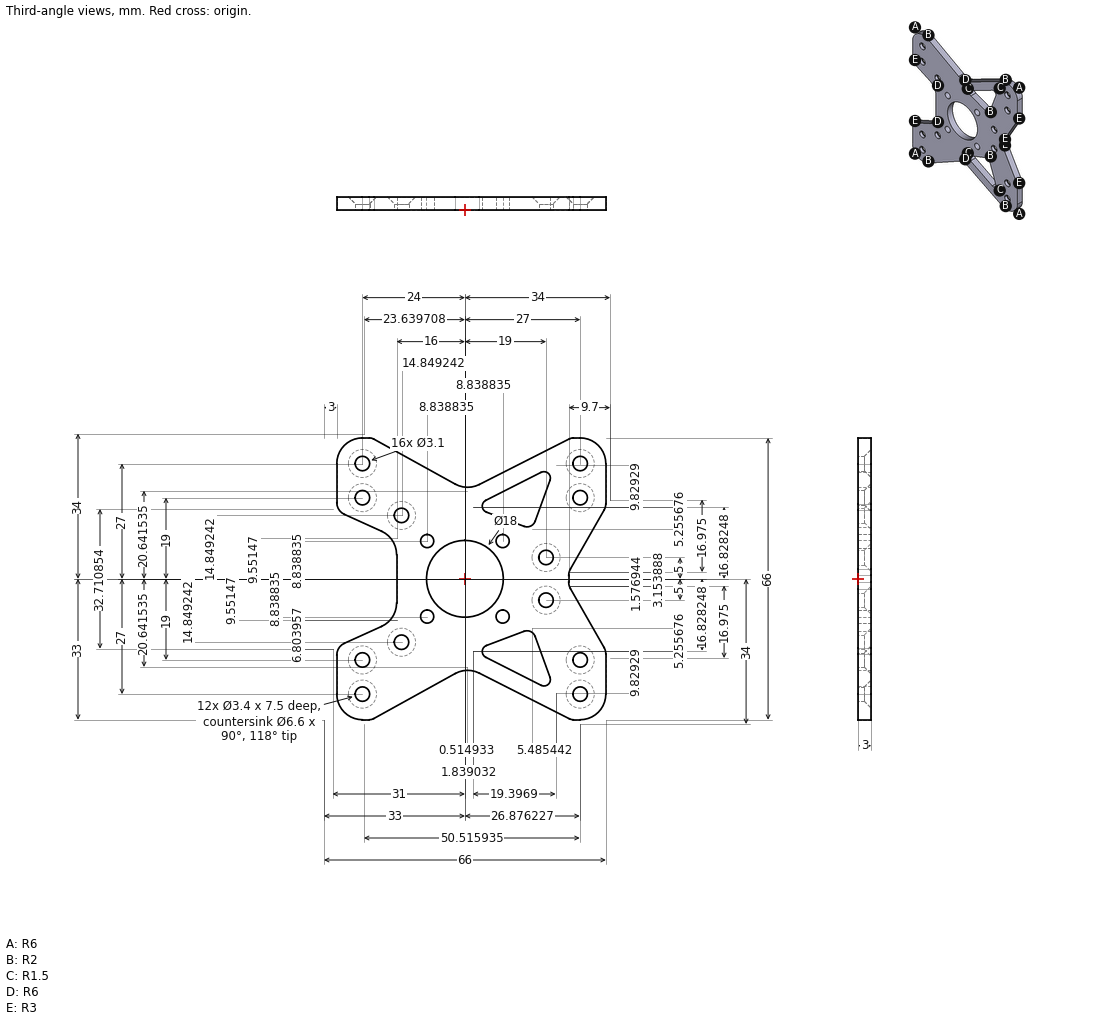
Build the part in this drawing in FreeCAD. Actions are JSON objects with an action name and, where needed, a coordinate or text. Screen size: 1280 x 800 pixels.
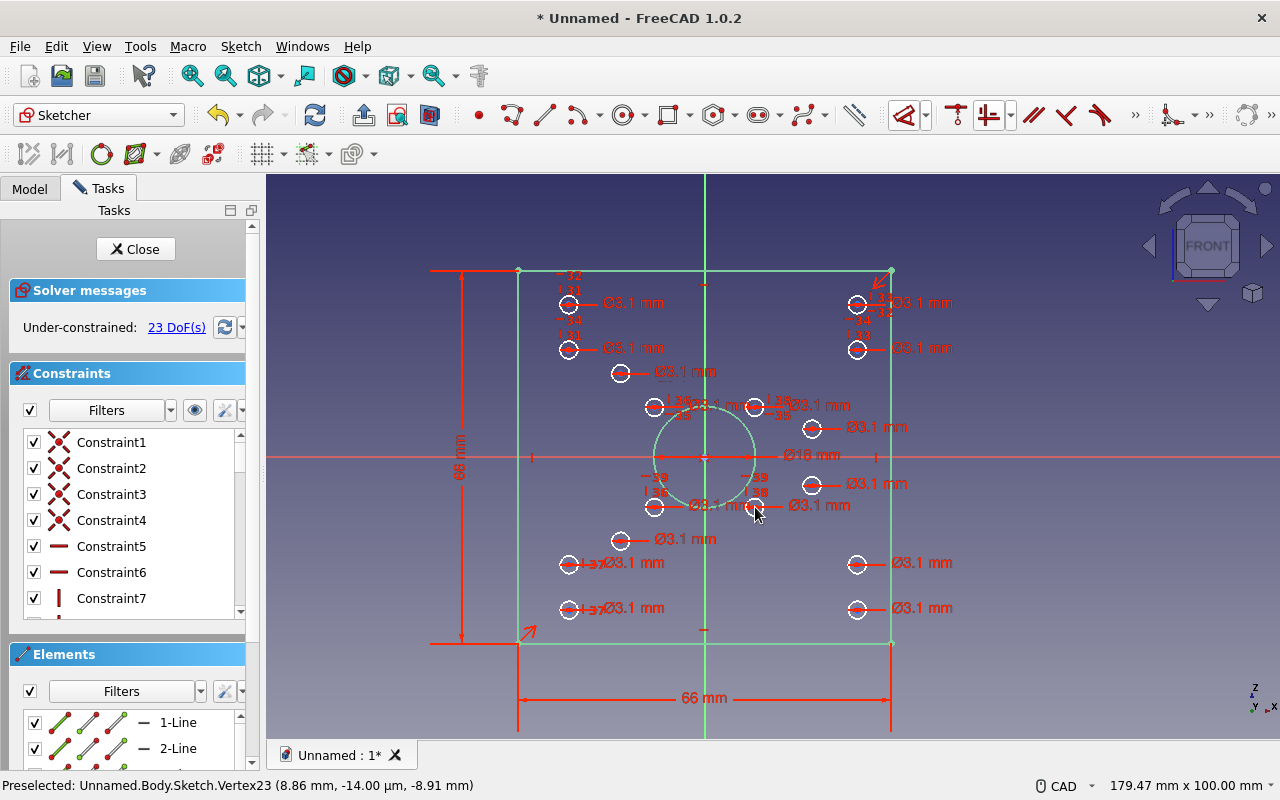
{"action": "left_click", "coordinate": [812, 429]}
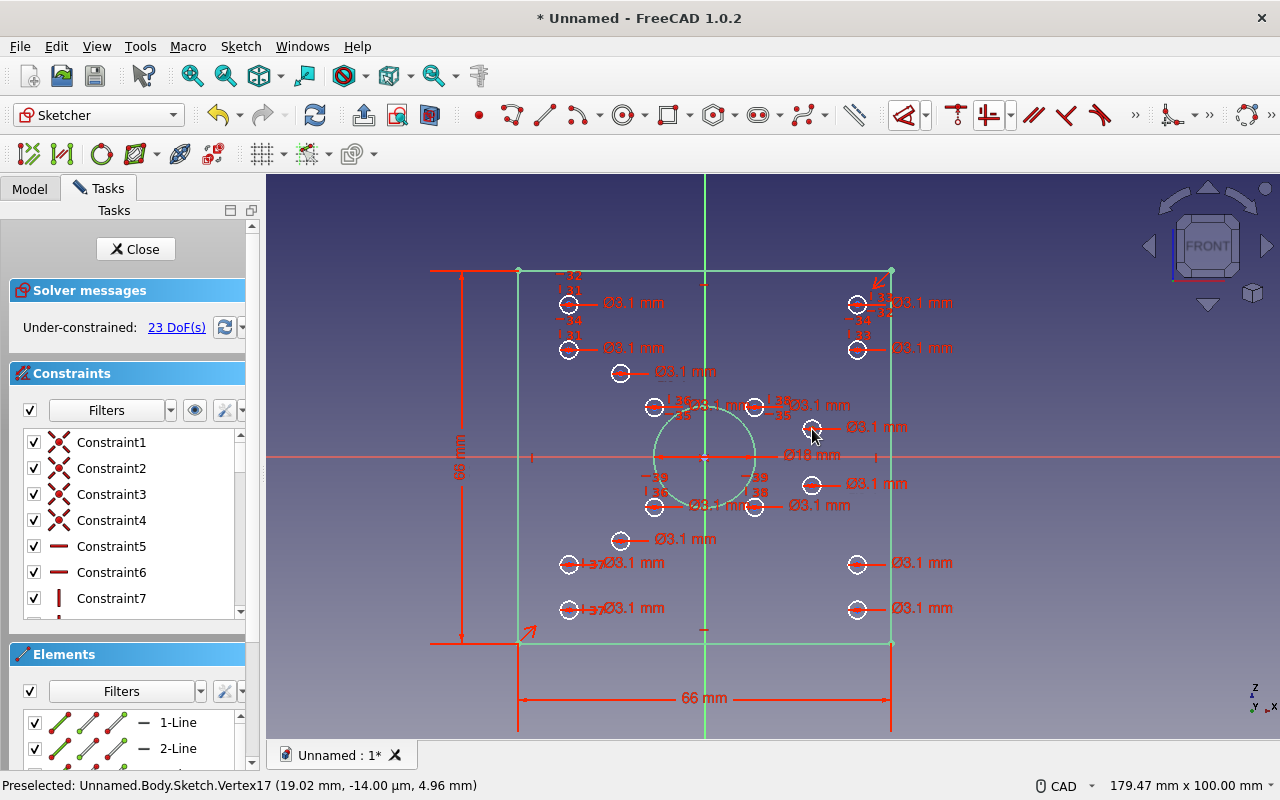
{"action": "left_click", "coordinate": [812, 486]}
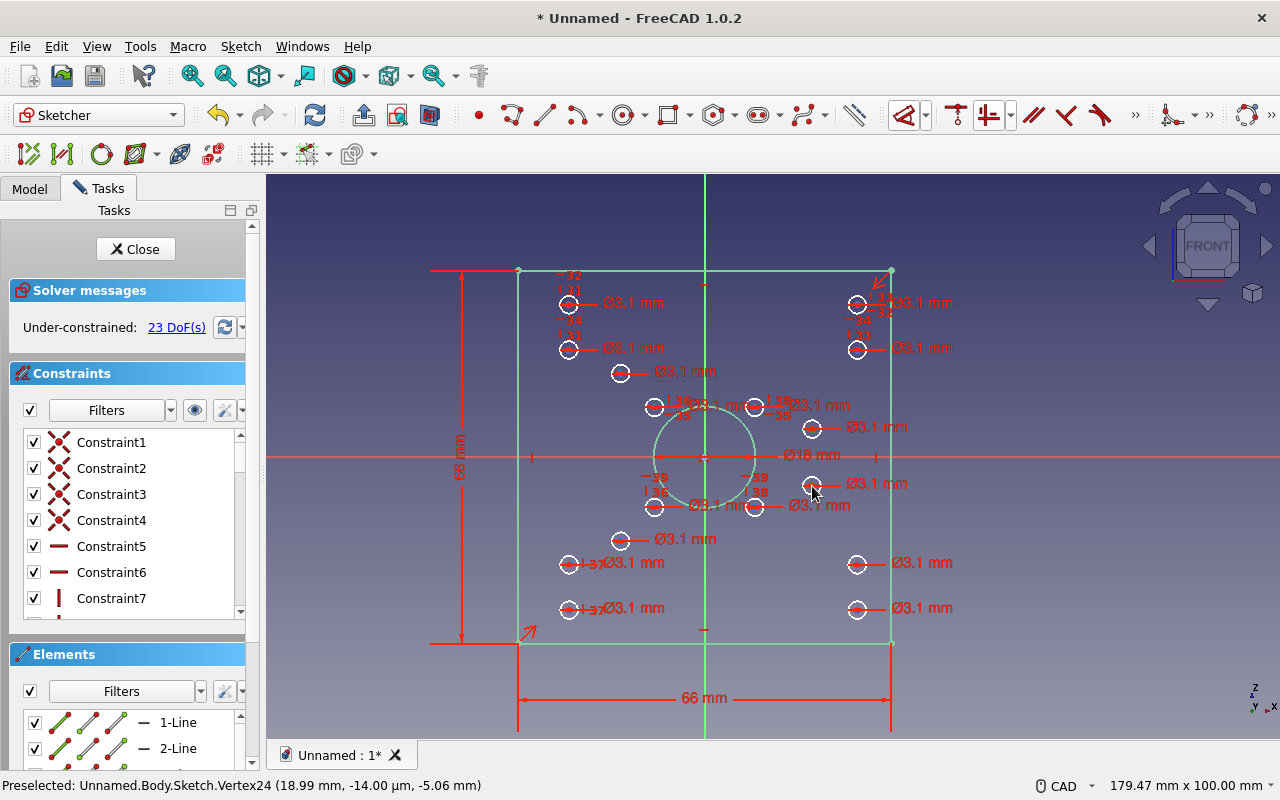
{"action": "key", "text": "v"}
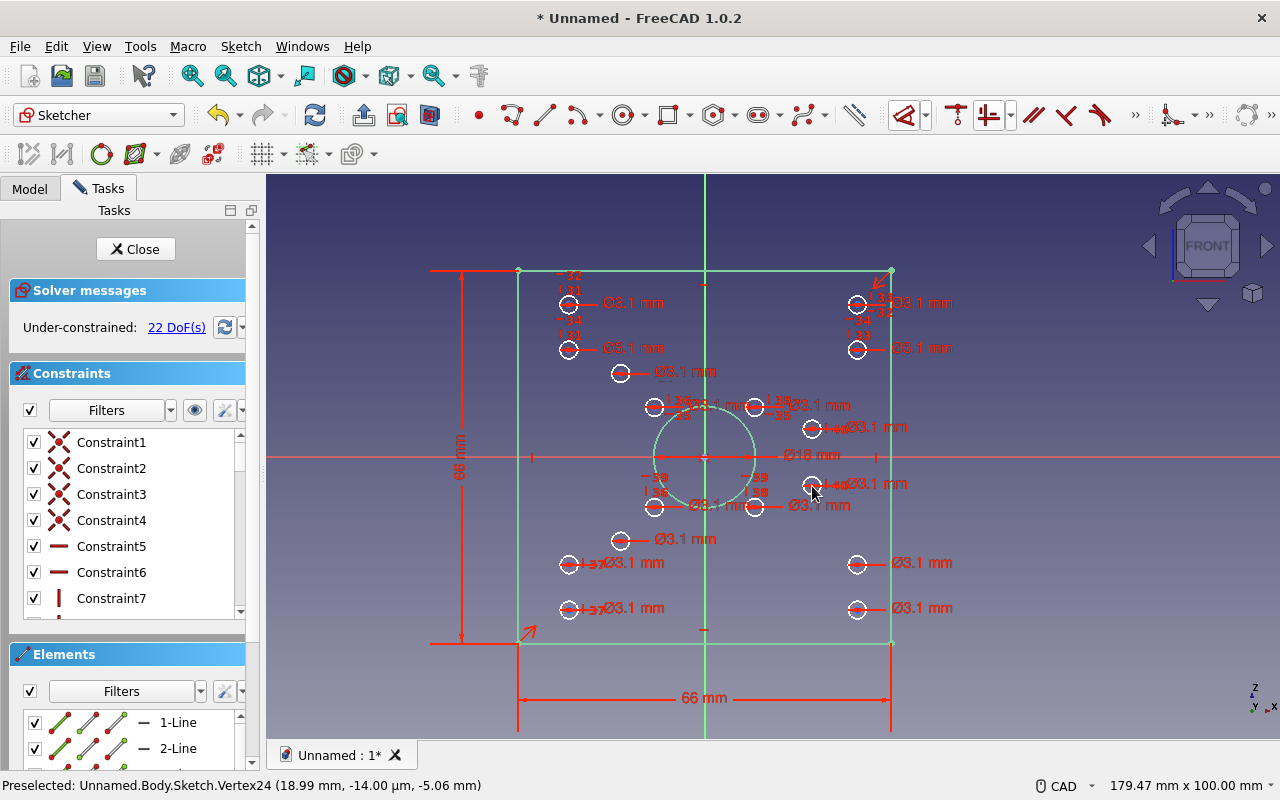
{"action": "left_click", "coordinate": [857, 565]}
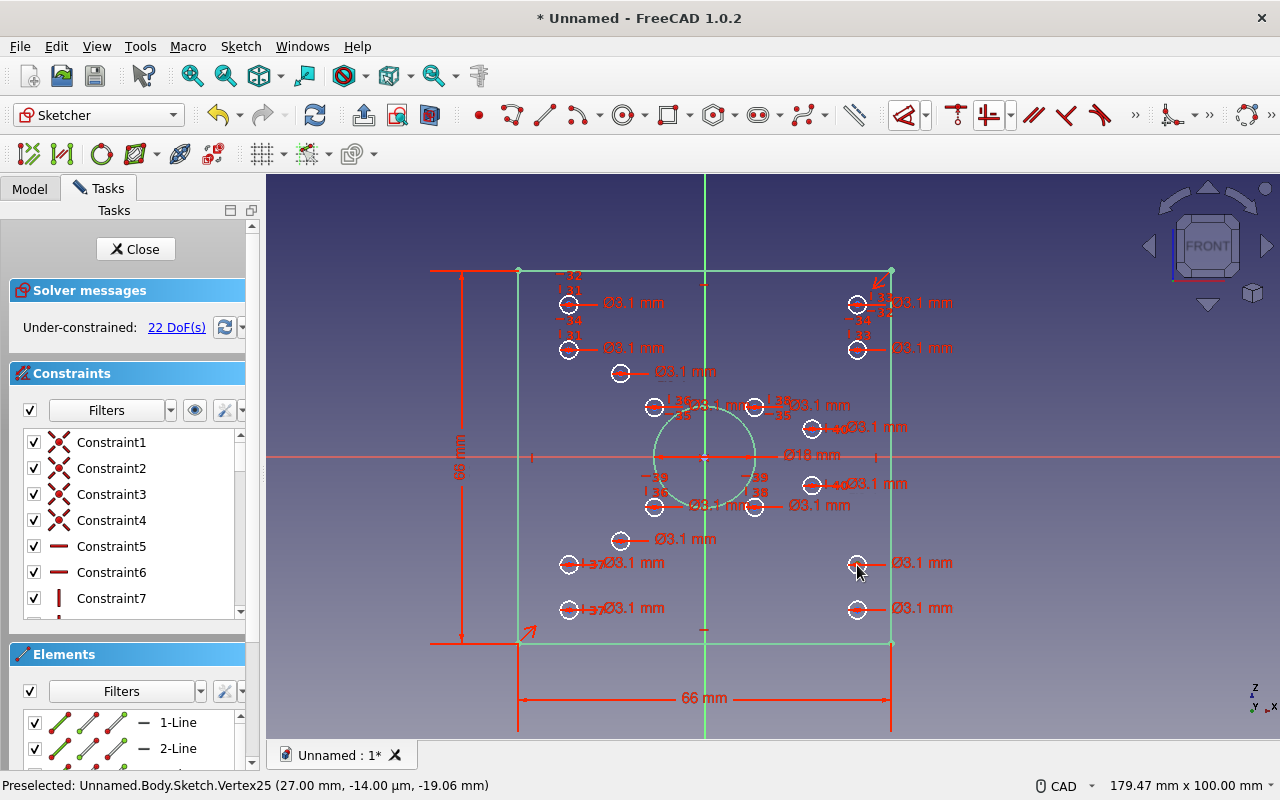
{"action": "left_click", "coordinate": [857, 610]}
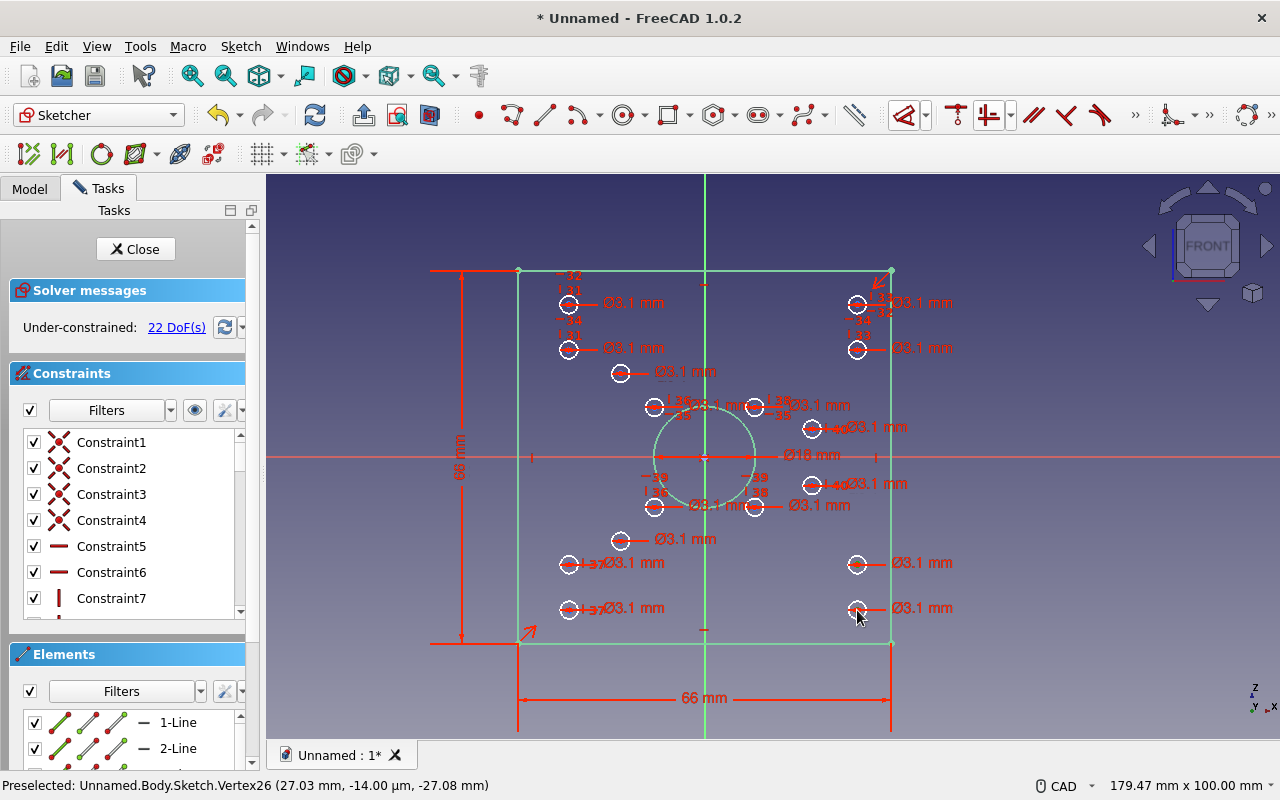
{"action": "key", "text": "v"}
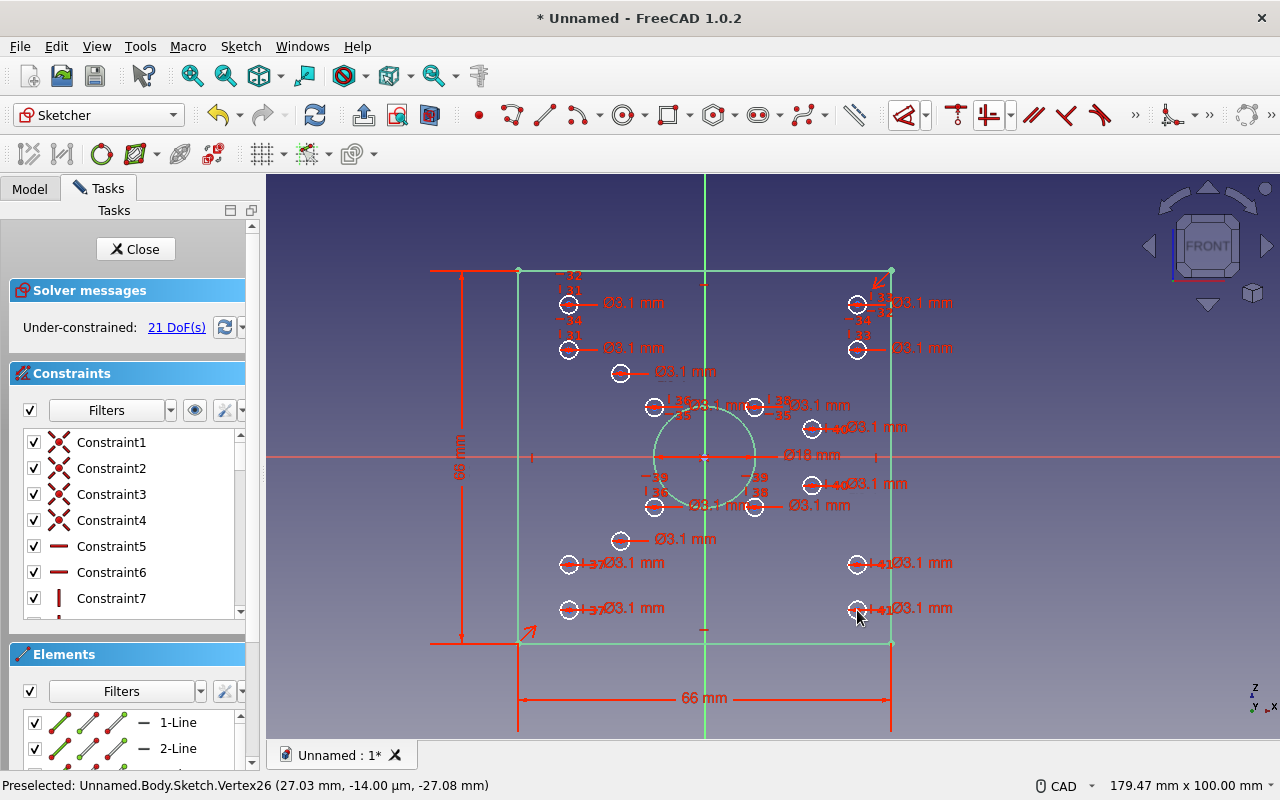
{"action": "left_click", "coordinate": [904, 116]}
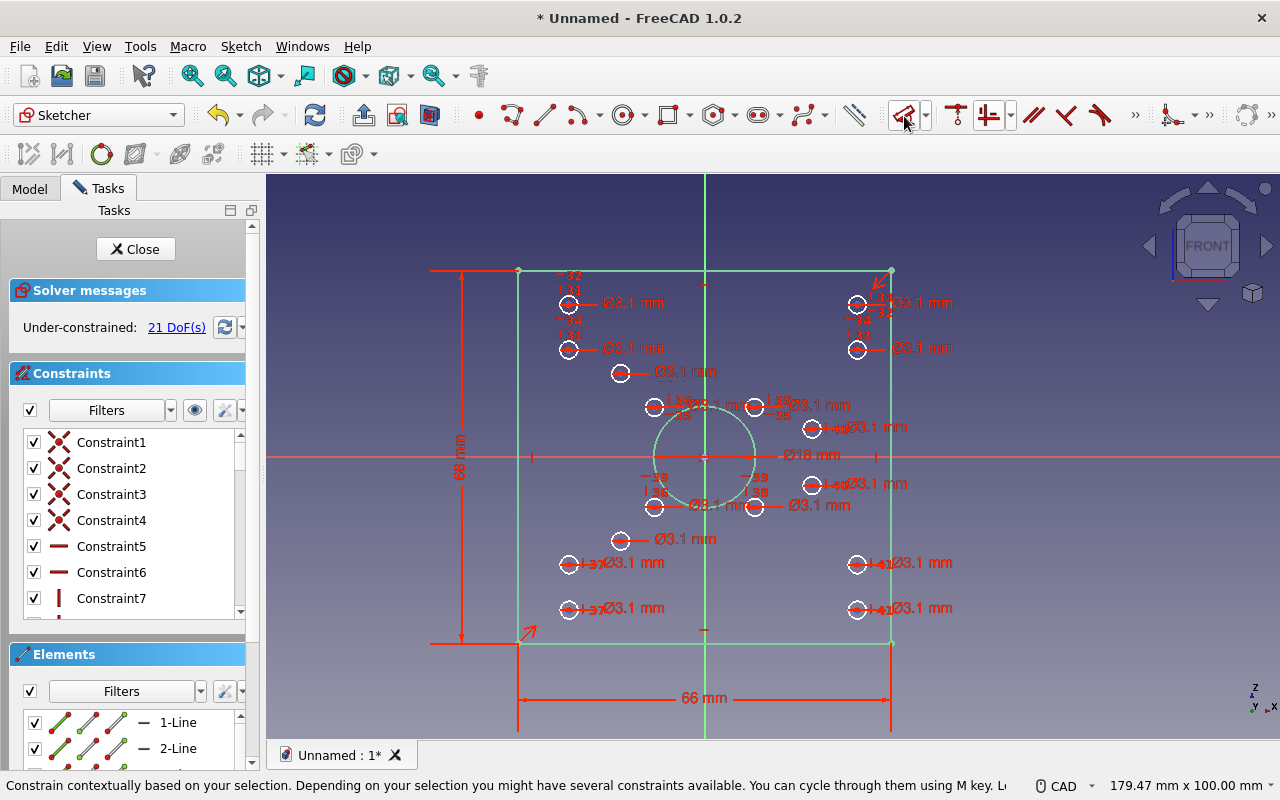
{"action": "scroll", "coordinate": [812, 429], "scroll_direction": "up", "scroll_amount": 2}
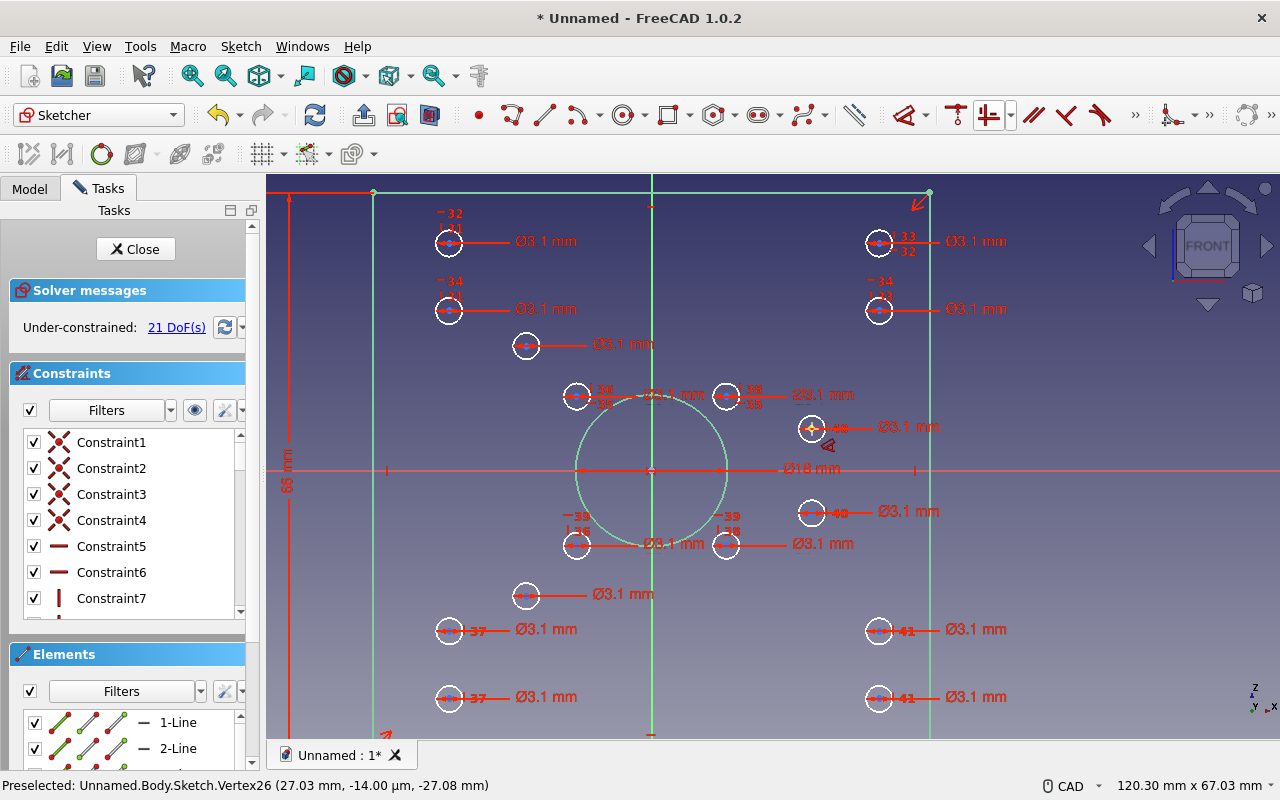
{"action": "left_click", "coordinate": [812, 429]}
{"action": "left_click", "coordinate": [846, 450]}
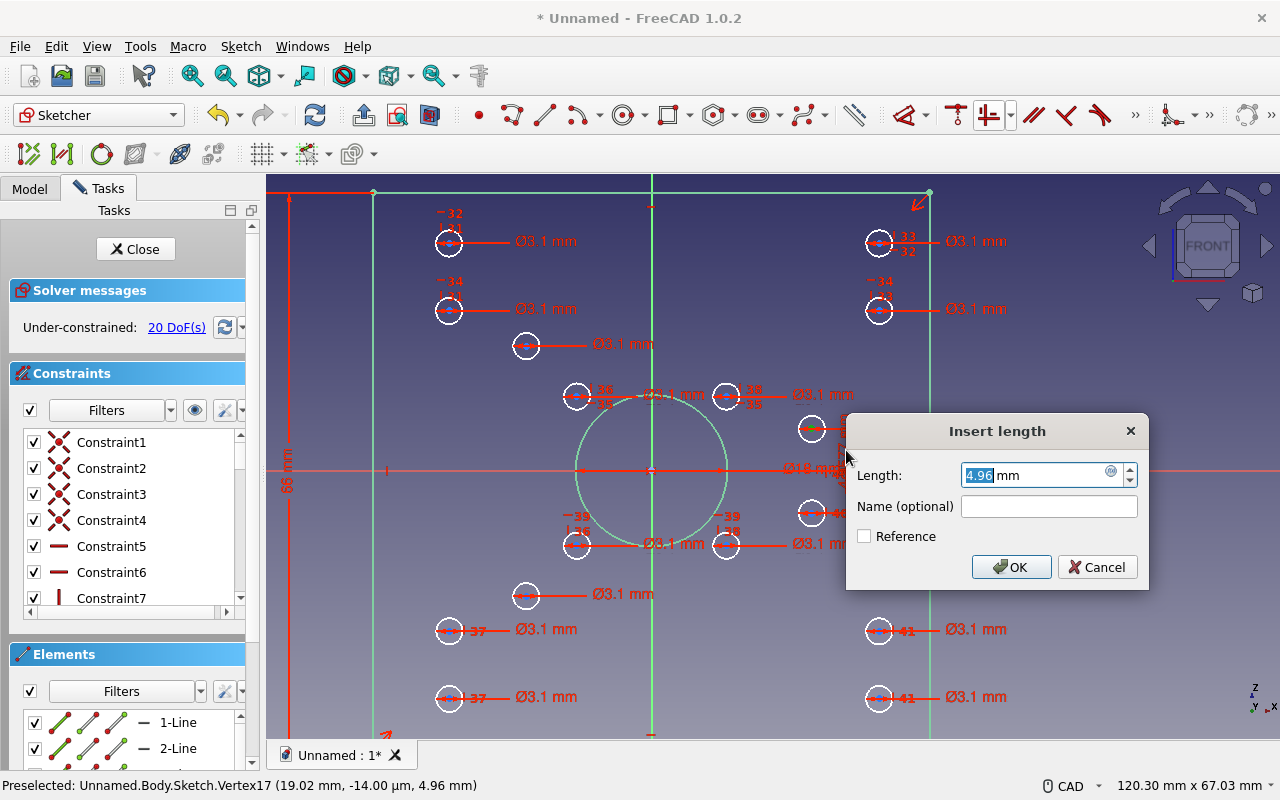
{"action": "type", "text": "5"}
{"action": "key", "text": "Return"}